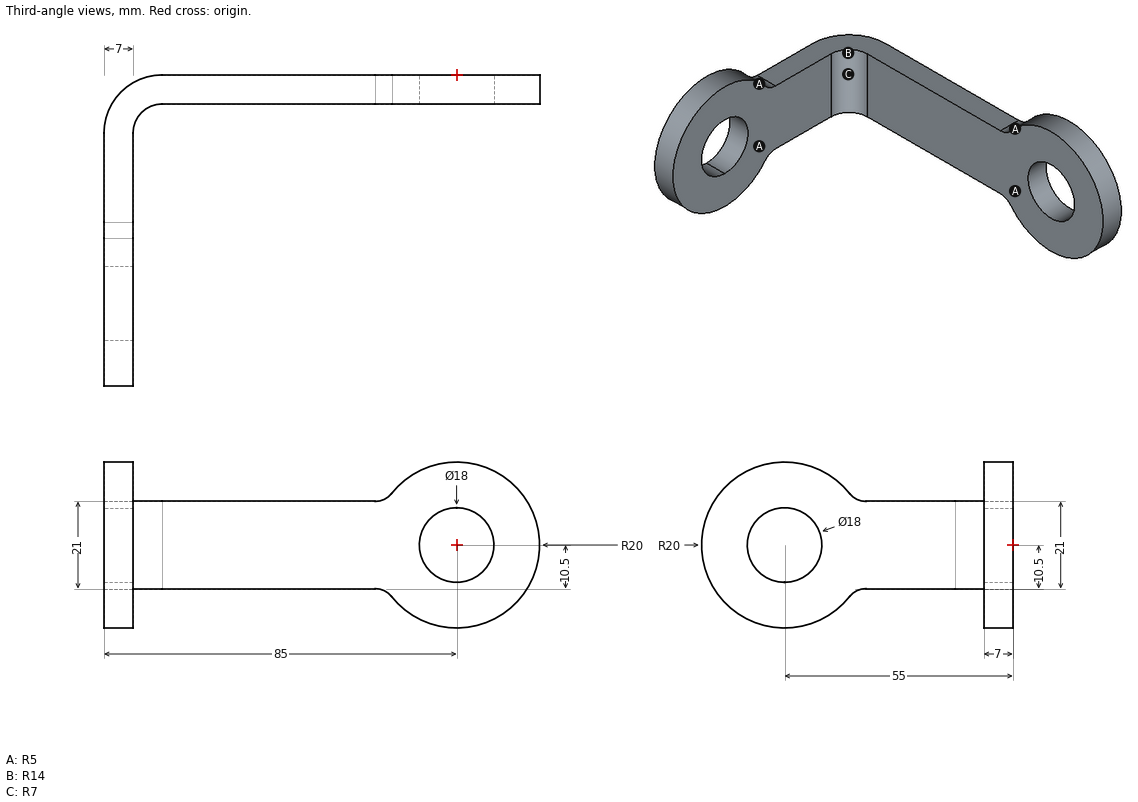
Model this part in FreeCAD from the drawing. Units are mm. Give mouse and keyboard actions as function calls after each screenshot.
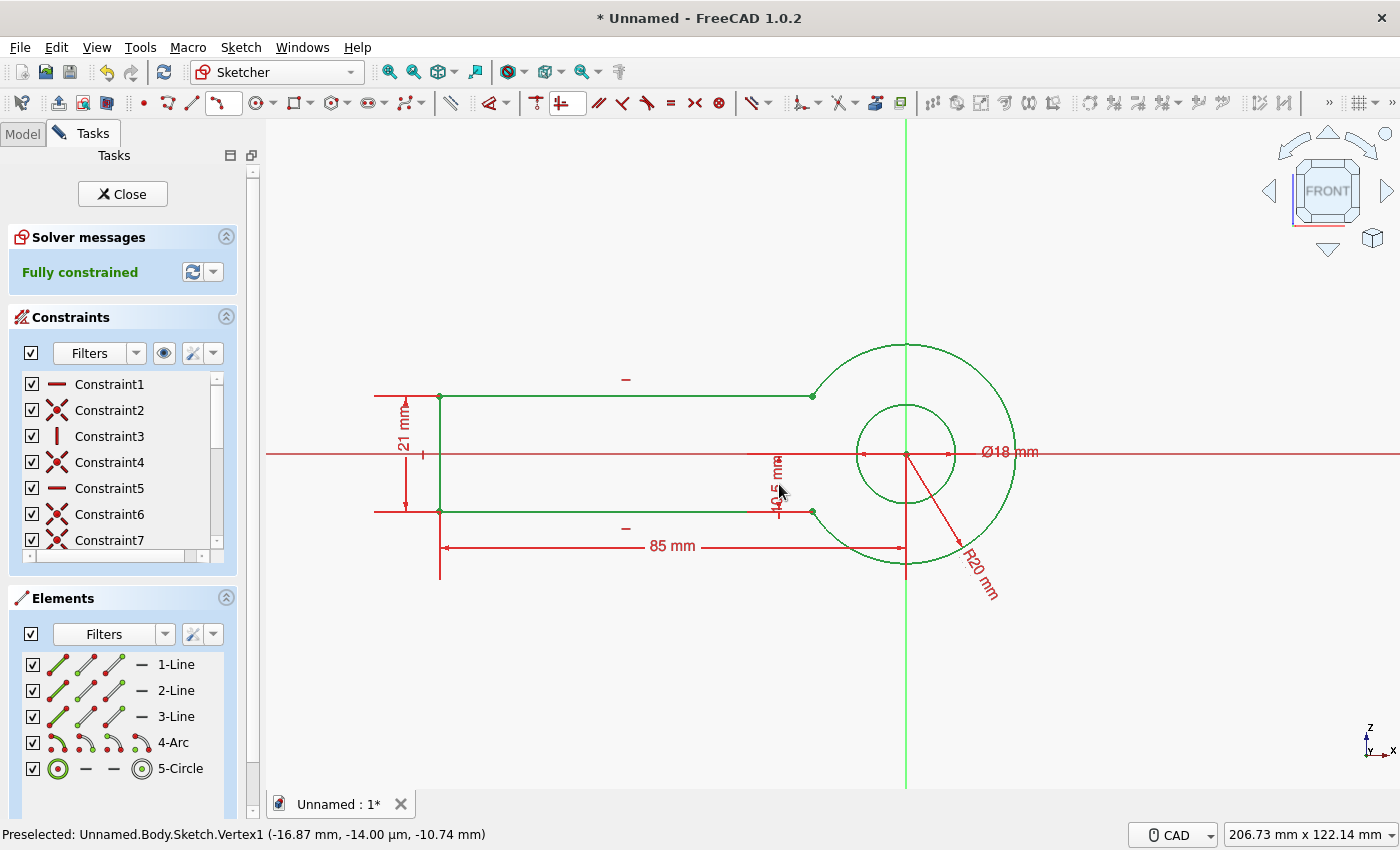
click(123, 194)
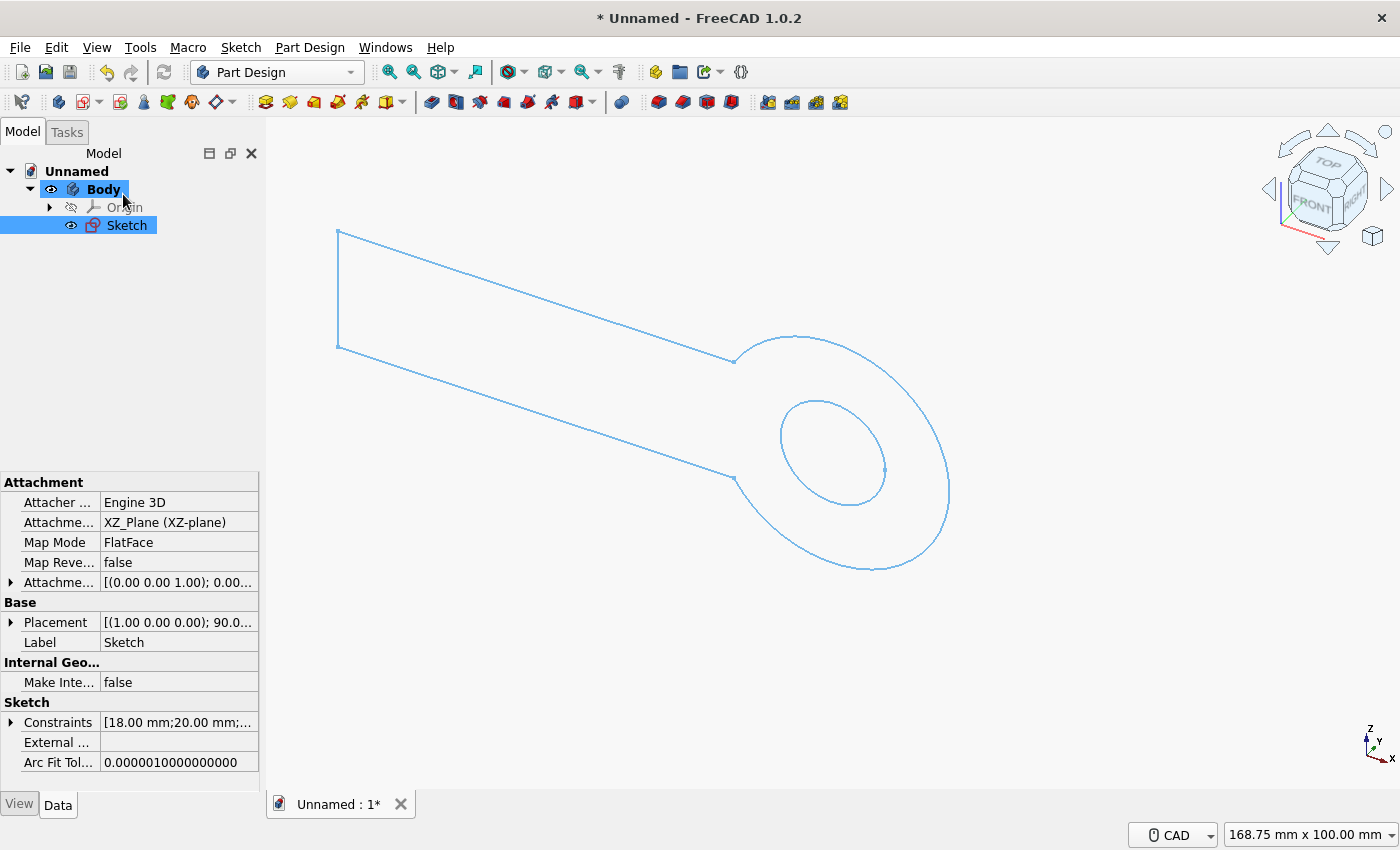
click(266, 102)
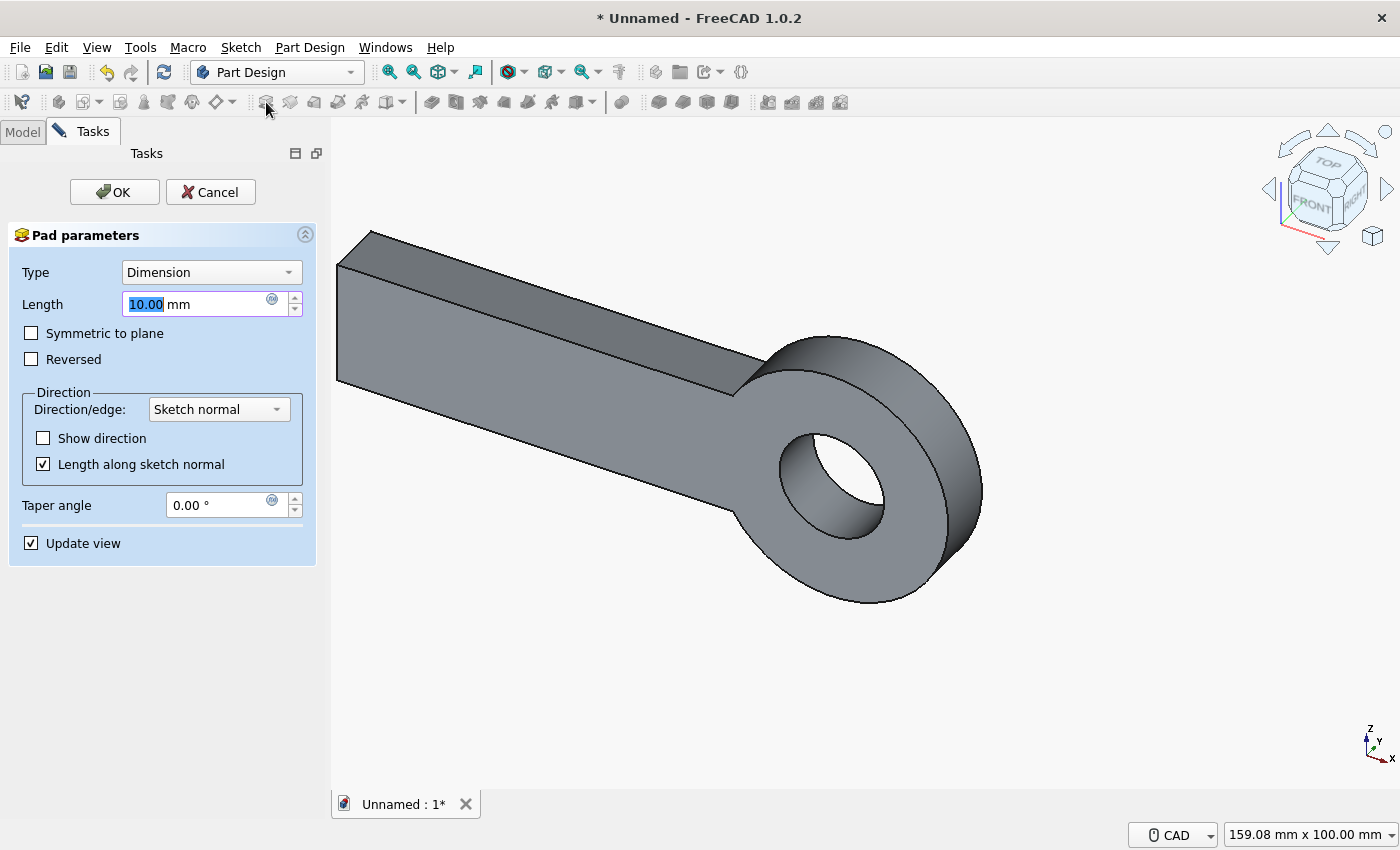
text(7)
key(Tab)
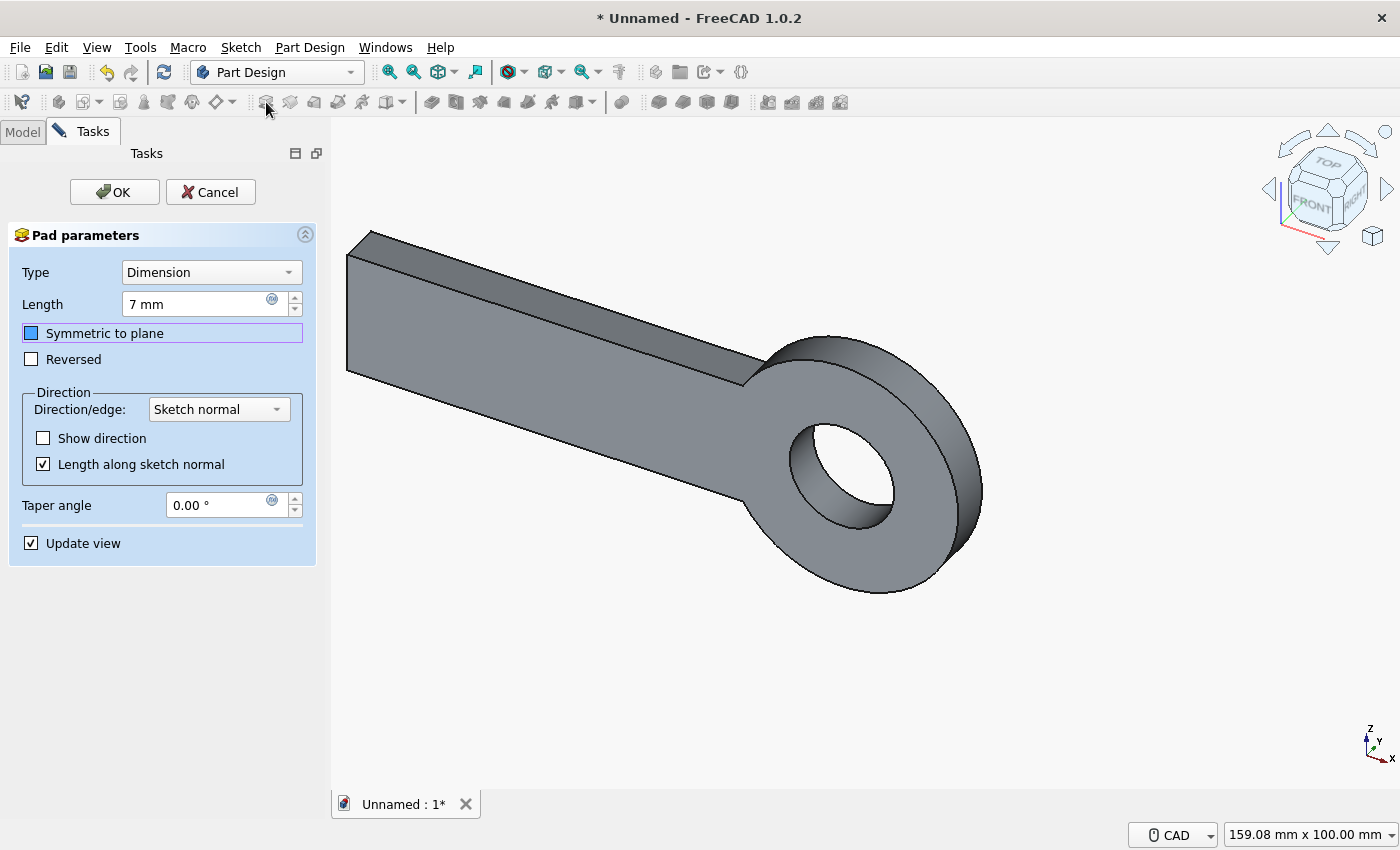
click(115, 192)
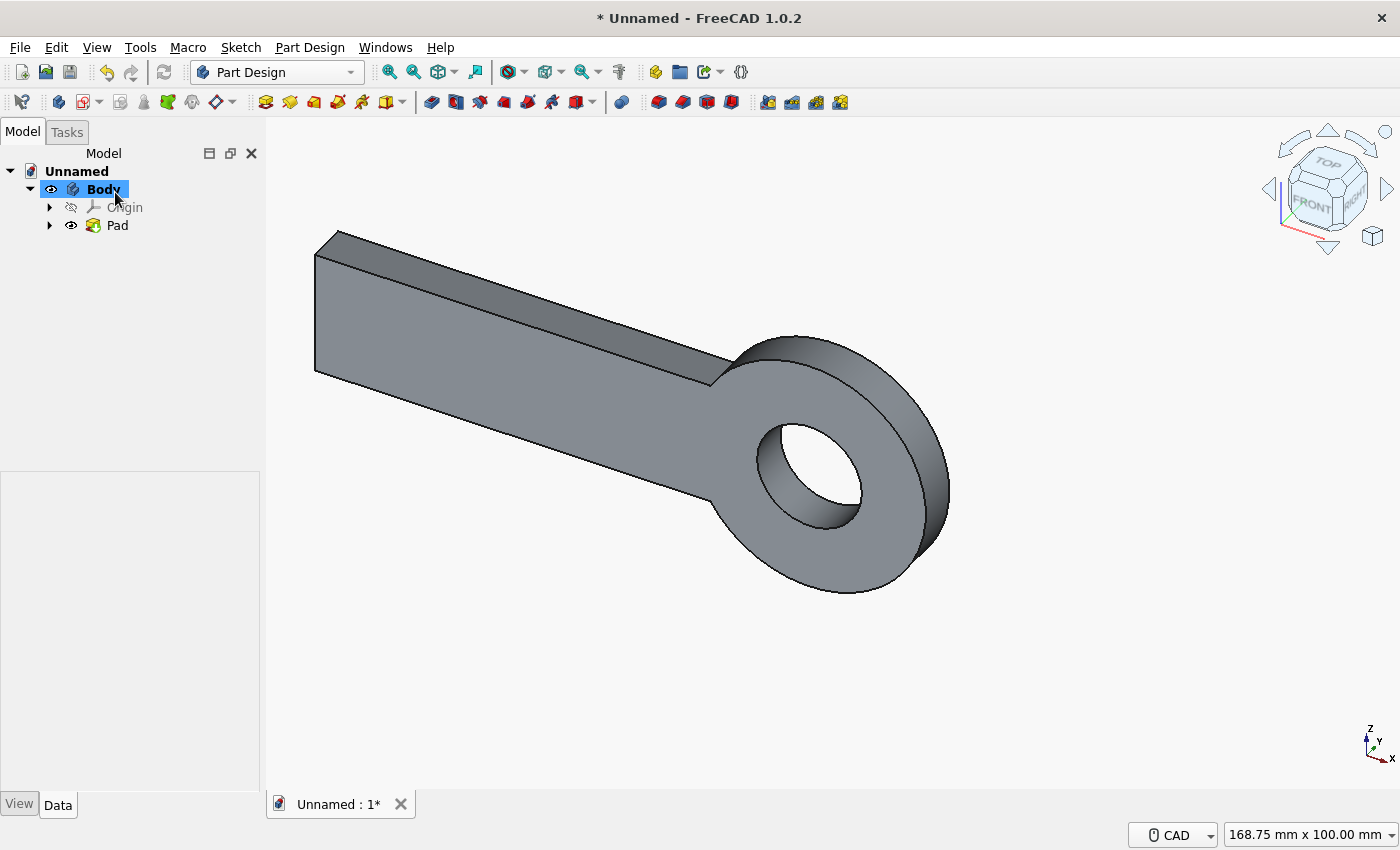
key(6)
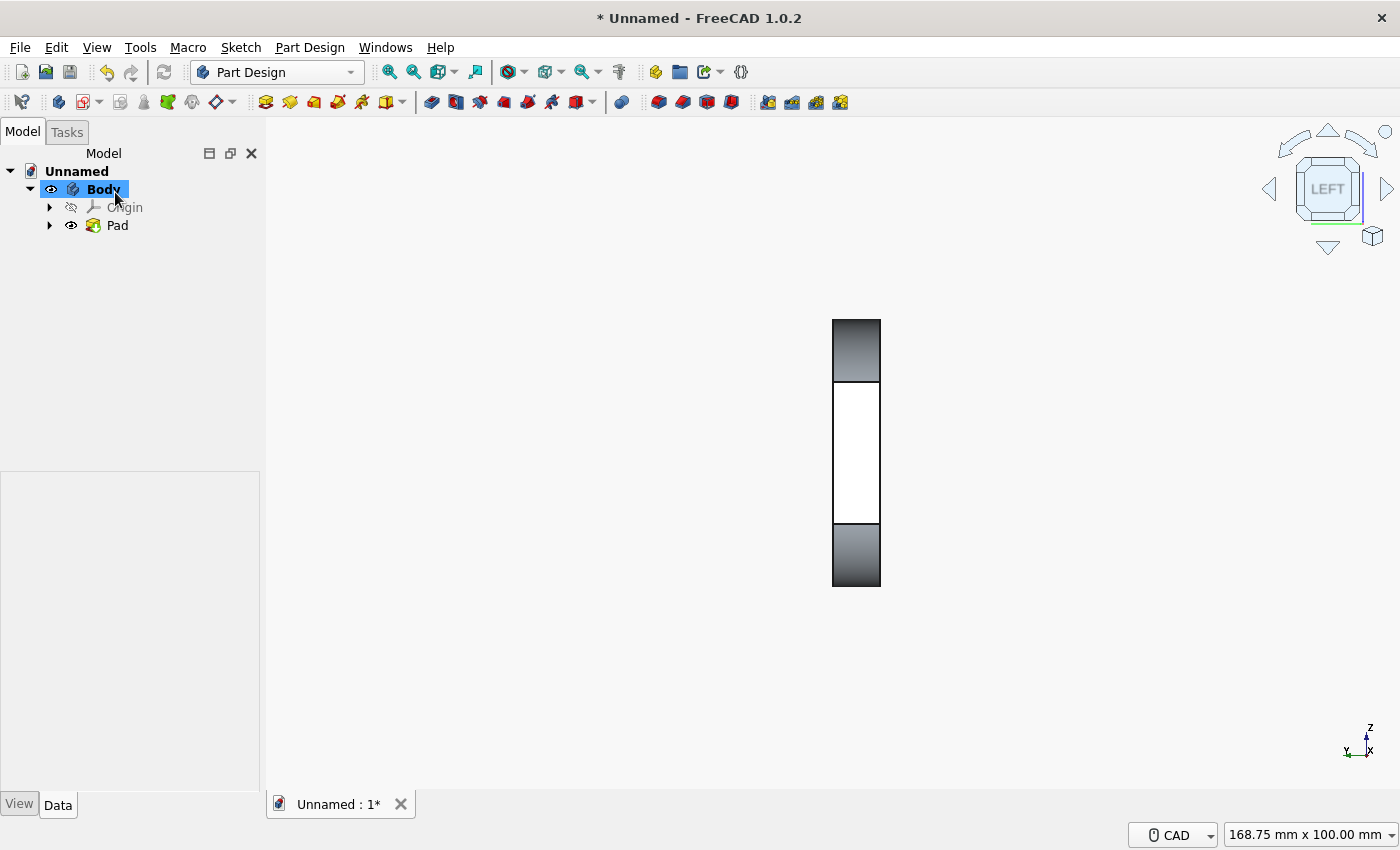
click(390, 72)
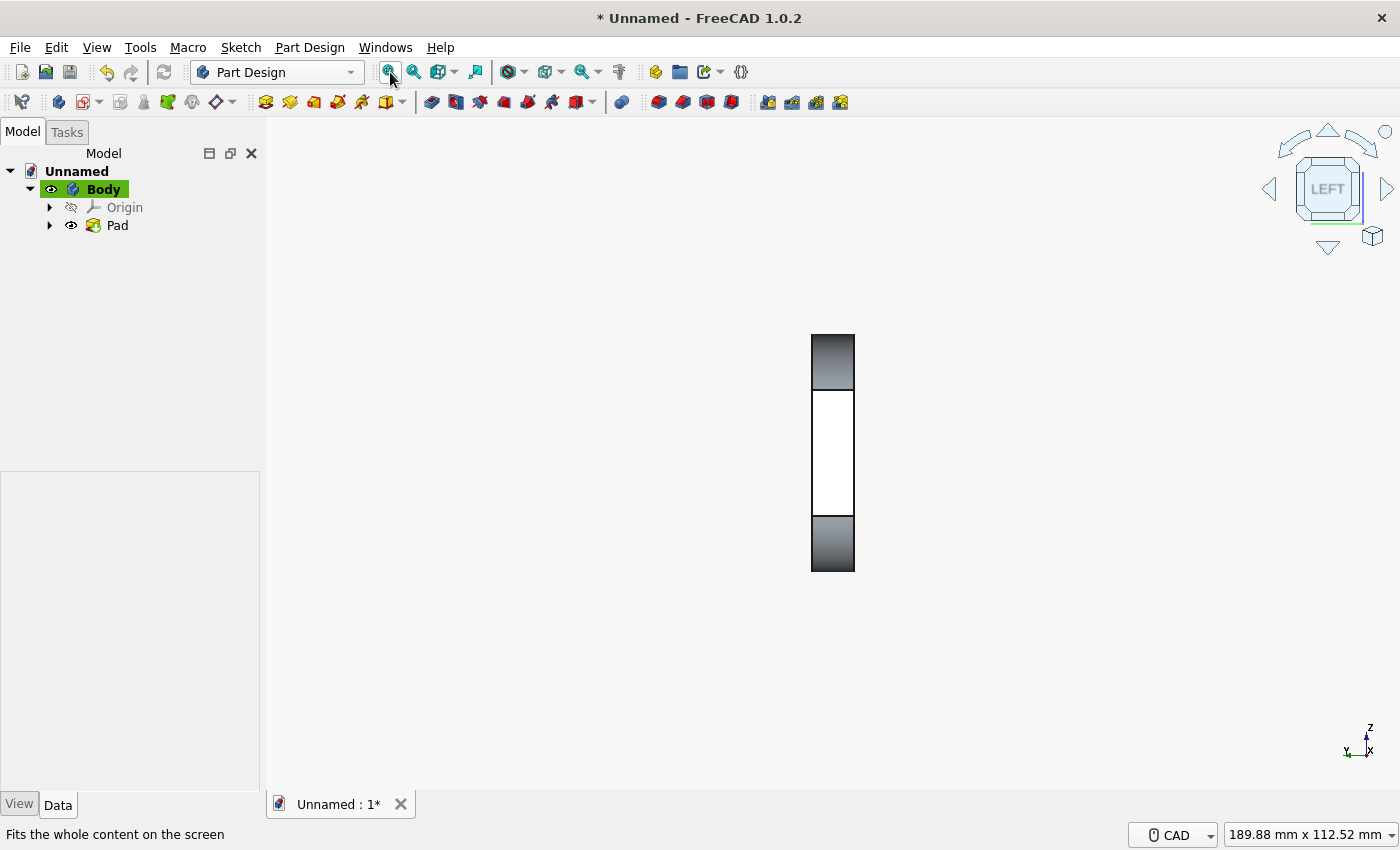
click(833, 416)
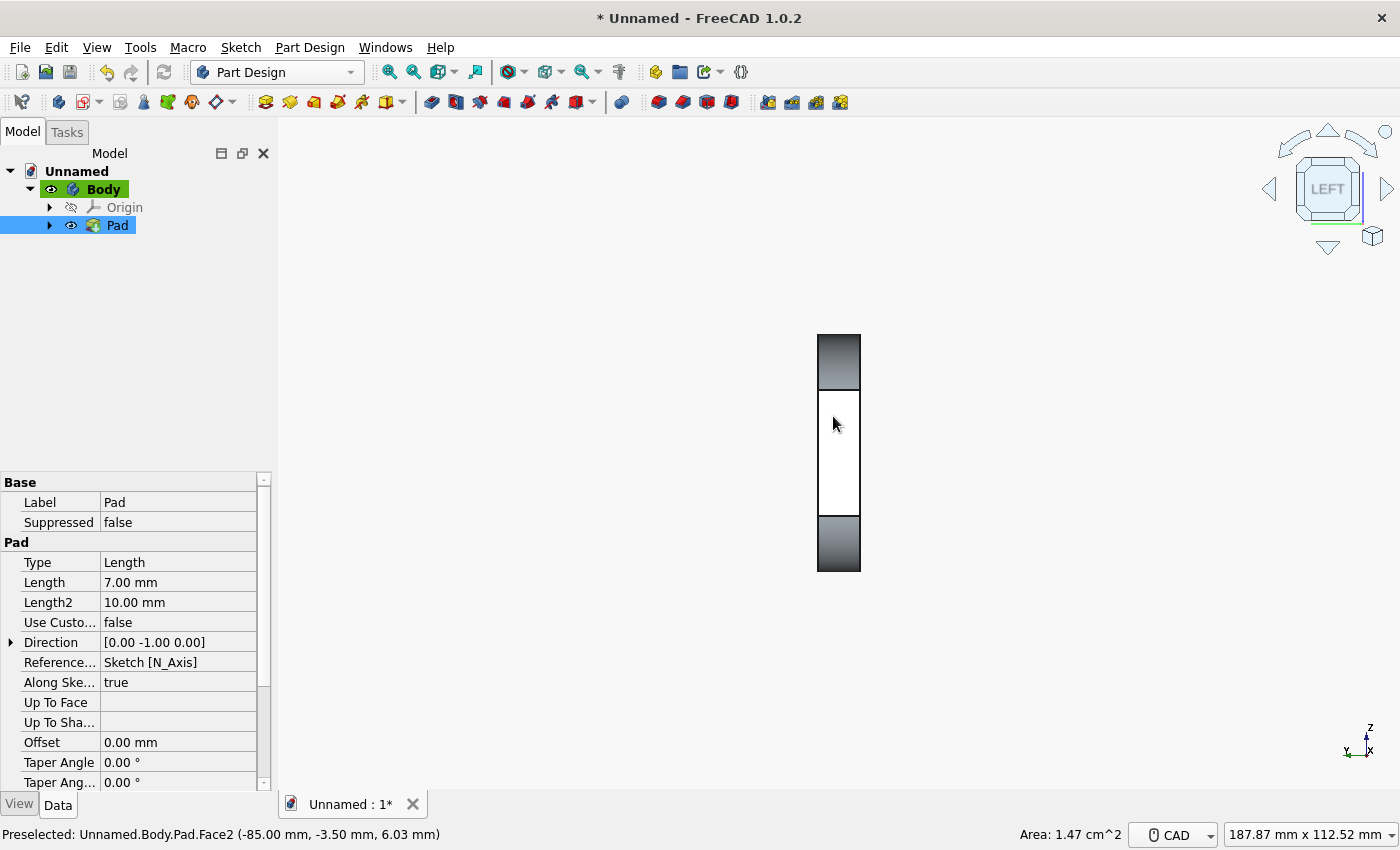
click(84, 102)